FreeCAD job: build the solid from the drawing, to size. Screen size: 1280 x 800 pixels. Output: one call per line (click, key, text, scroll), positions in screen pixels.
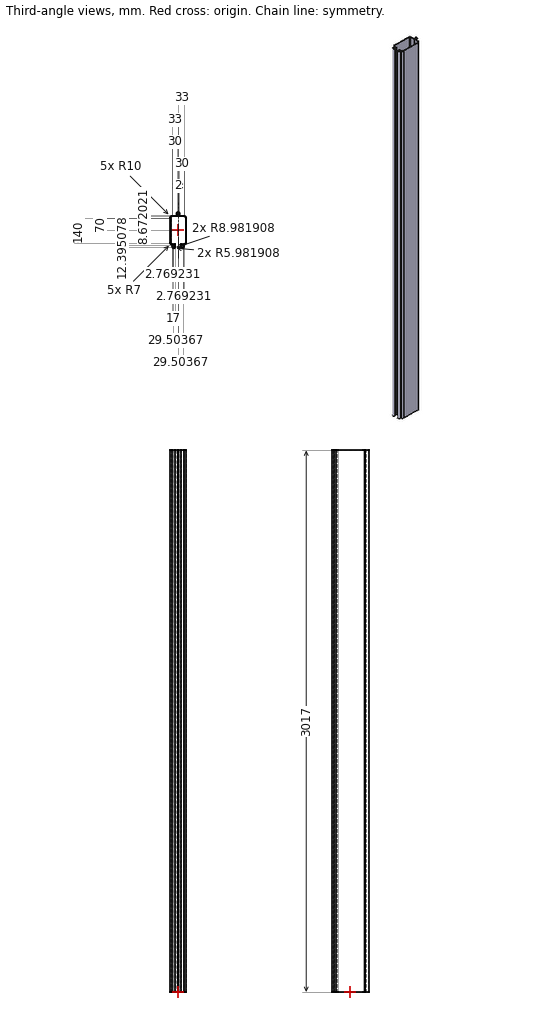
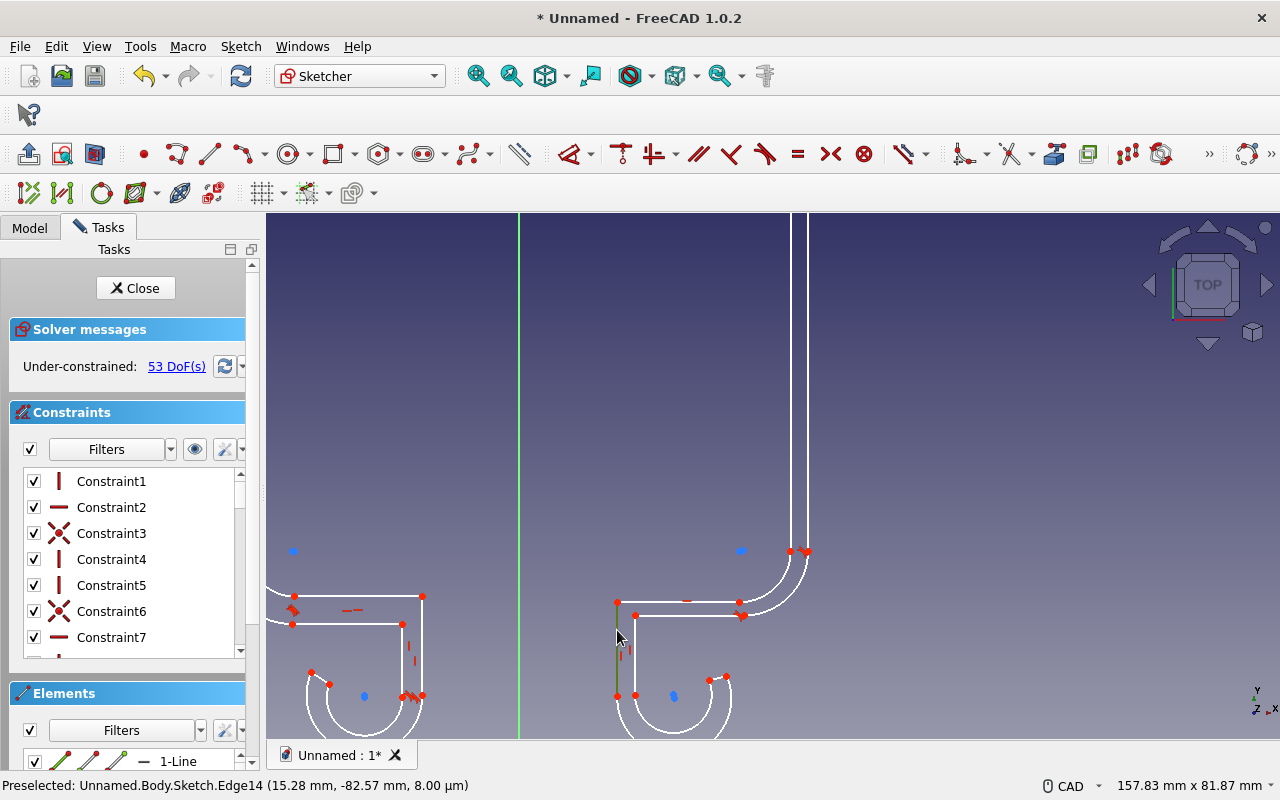
scroll(765, 600, down, 7)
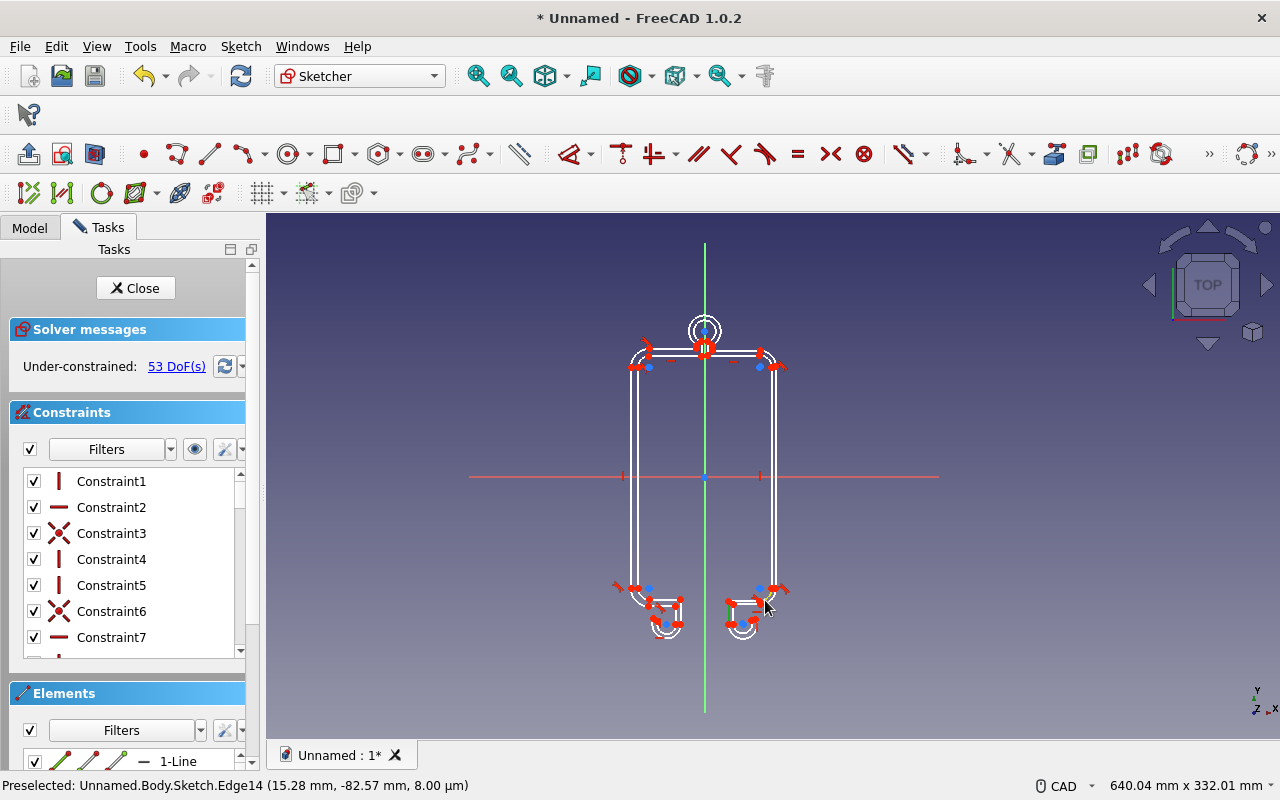
scroll(736, 637, up, 5)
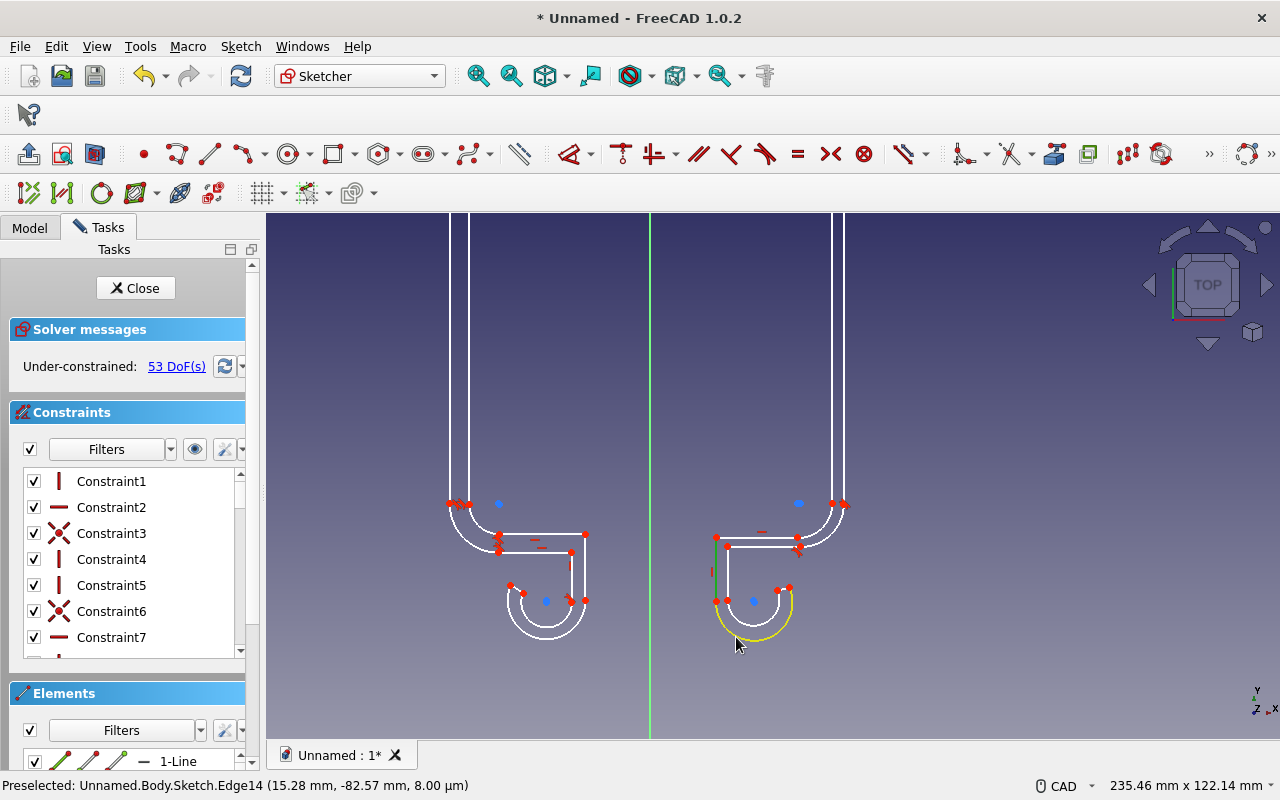
click(735, 635)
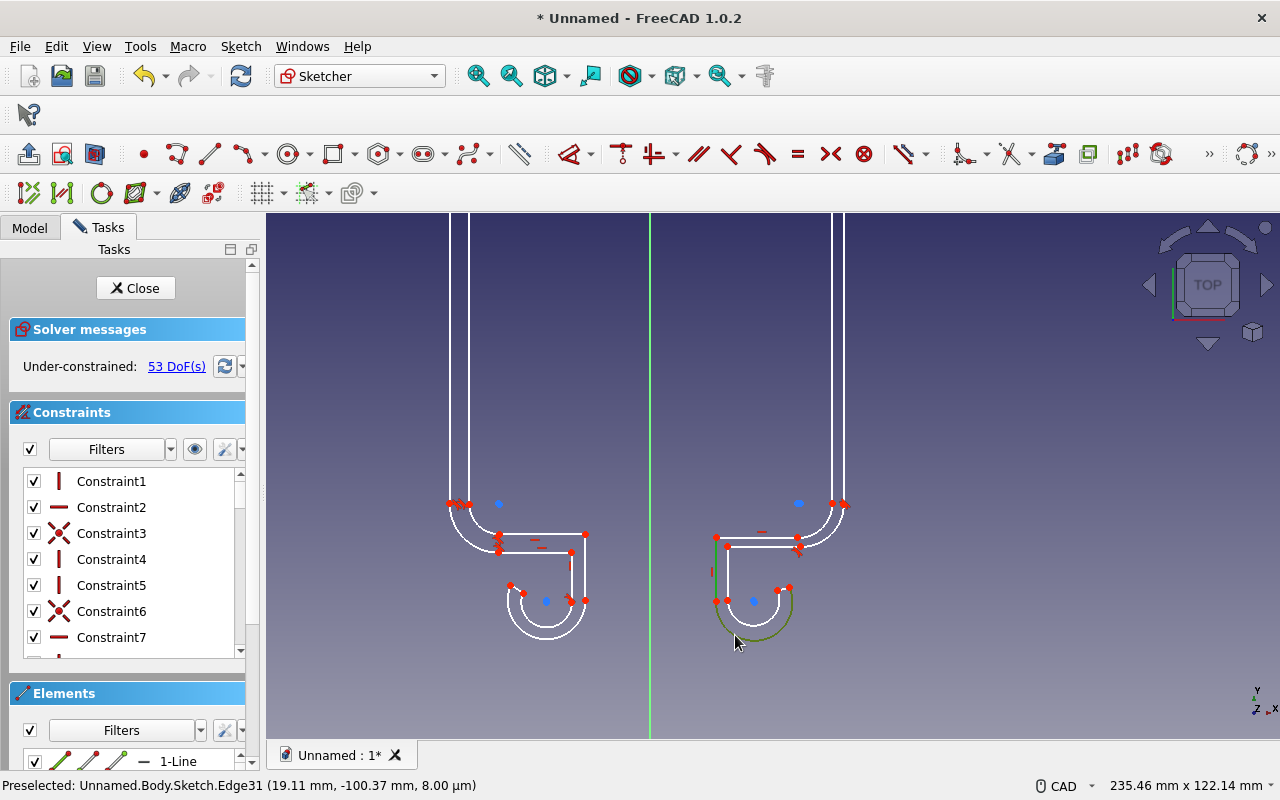
click(765, 154)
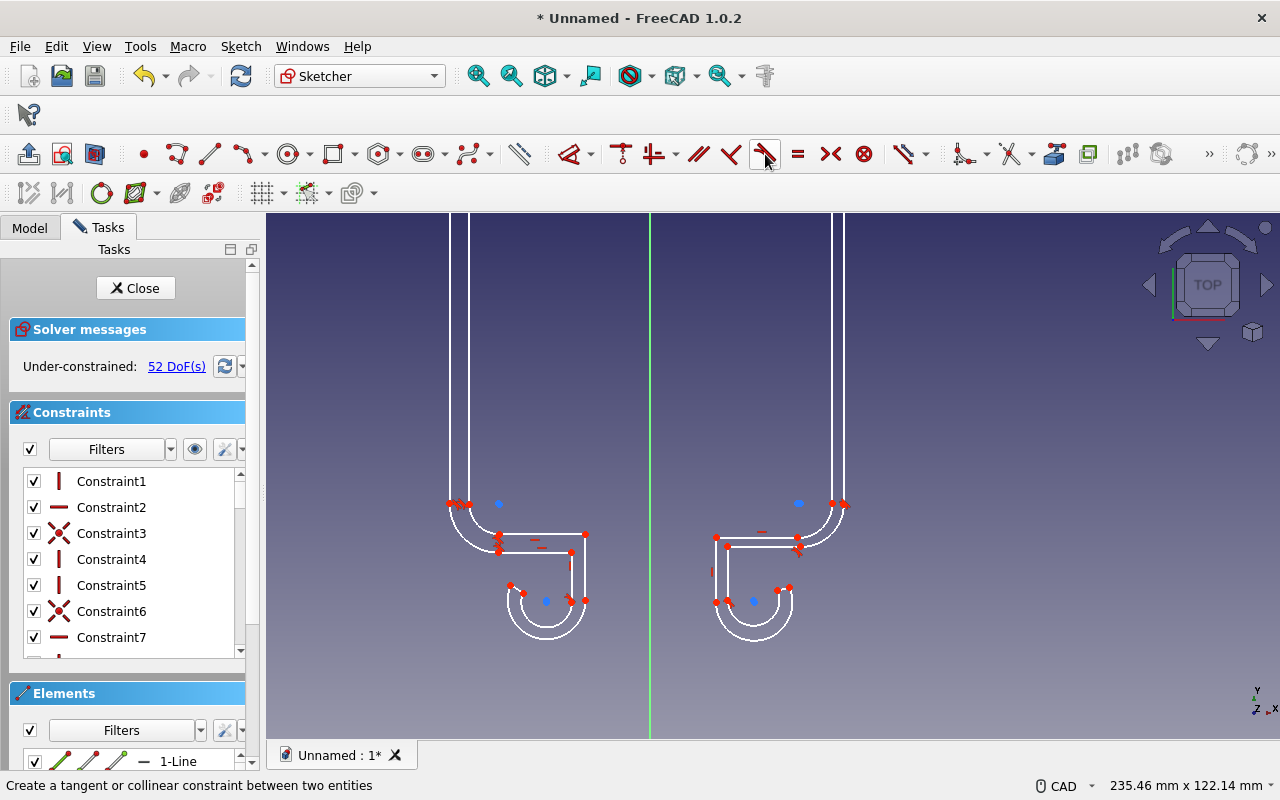
click(728, 585)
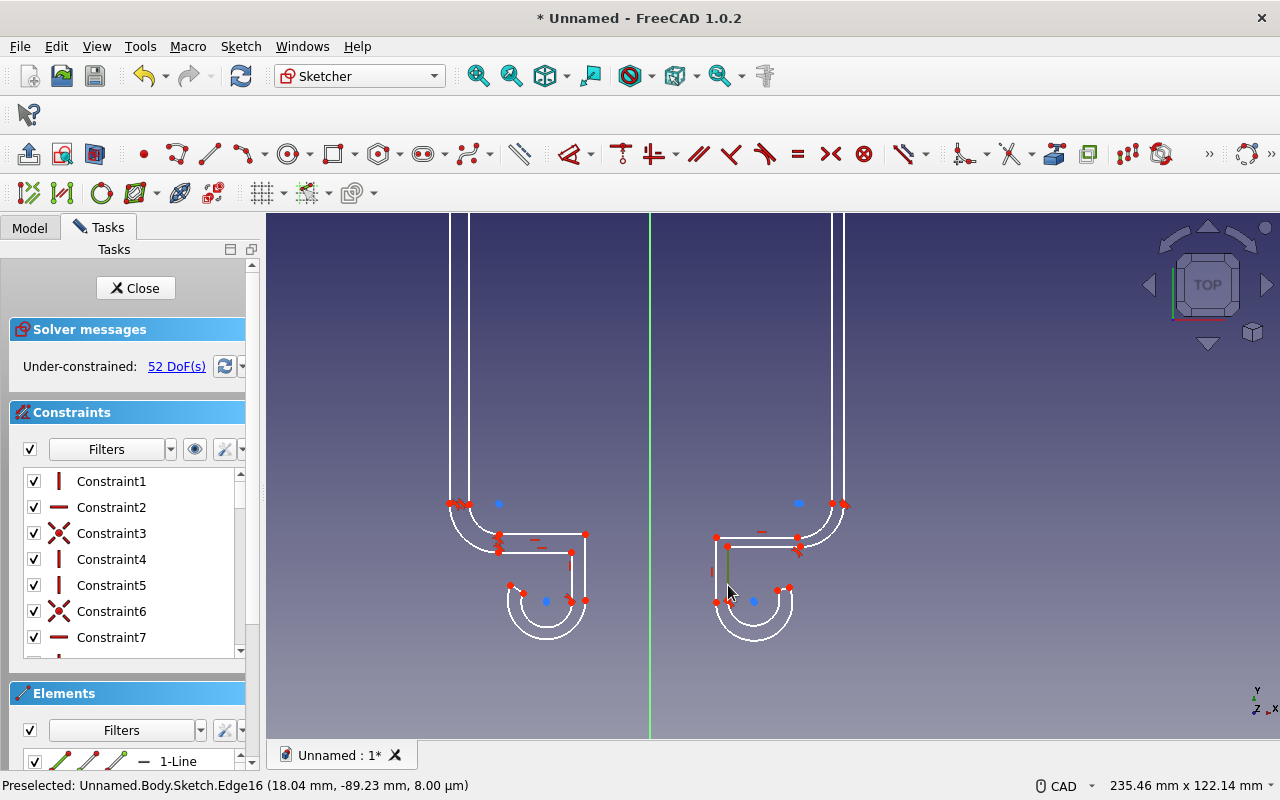
click(741, 623)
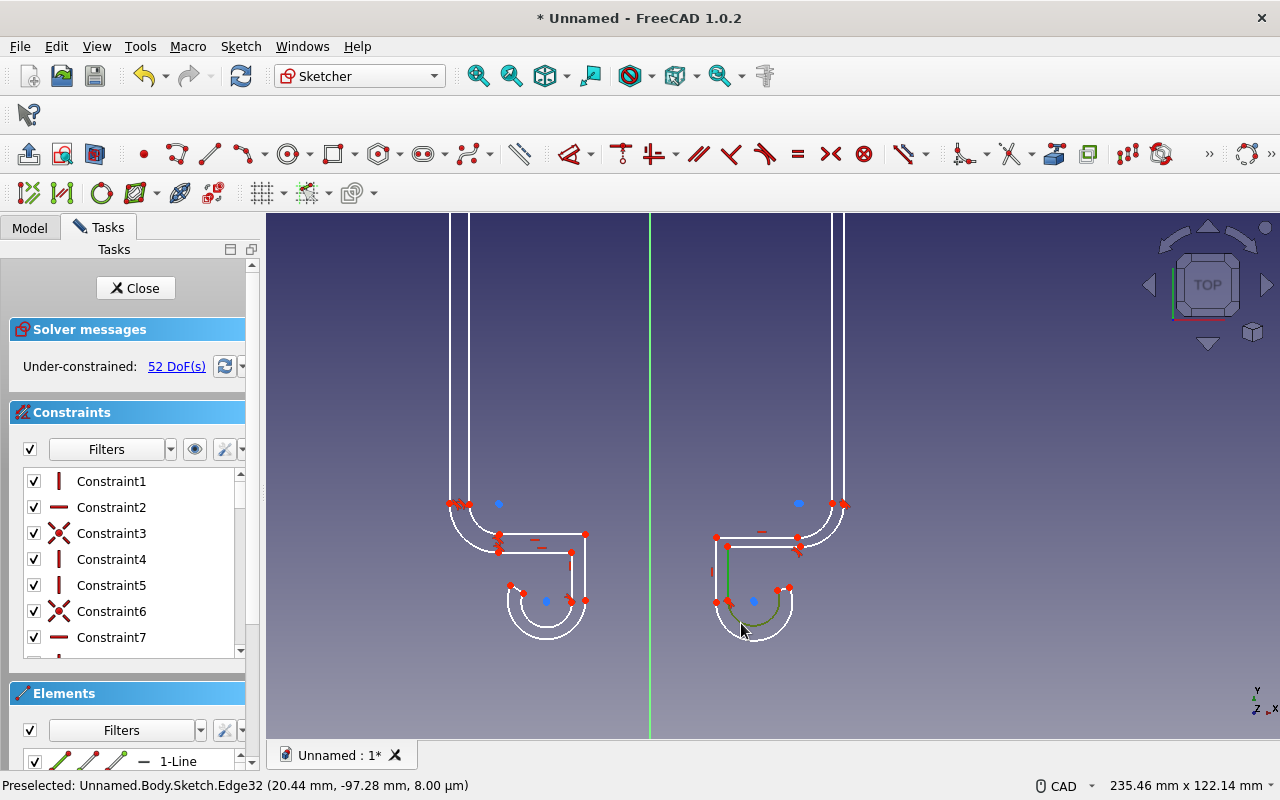
click(765, 154)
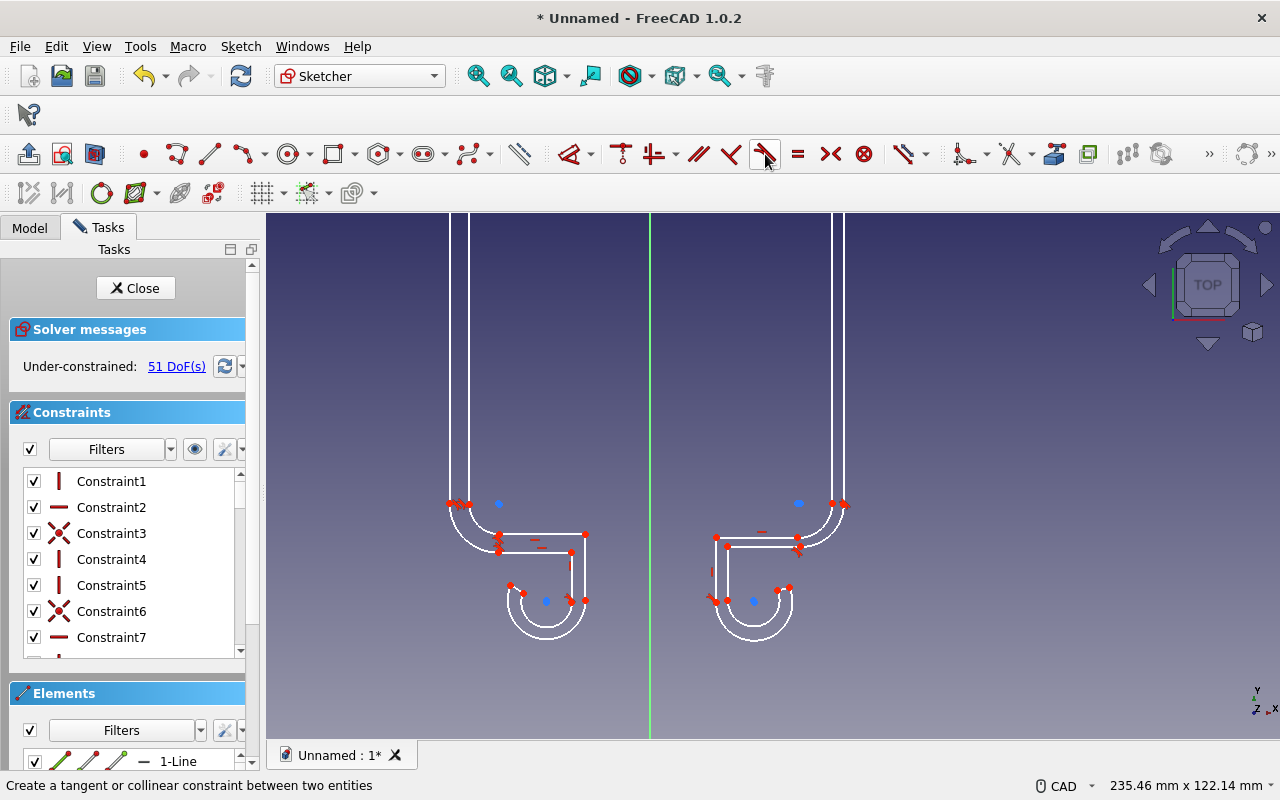
scroll(750, 547, up, 3)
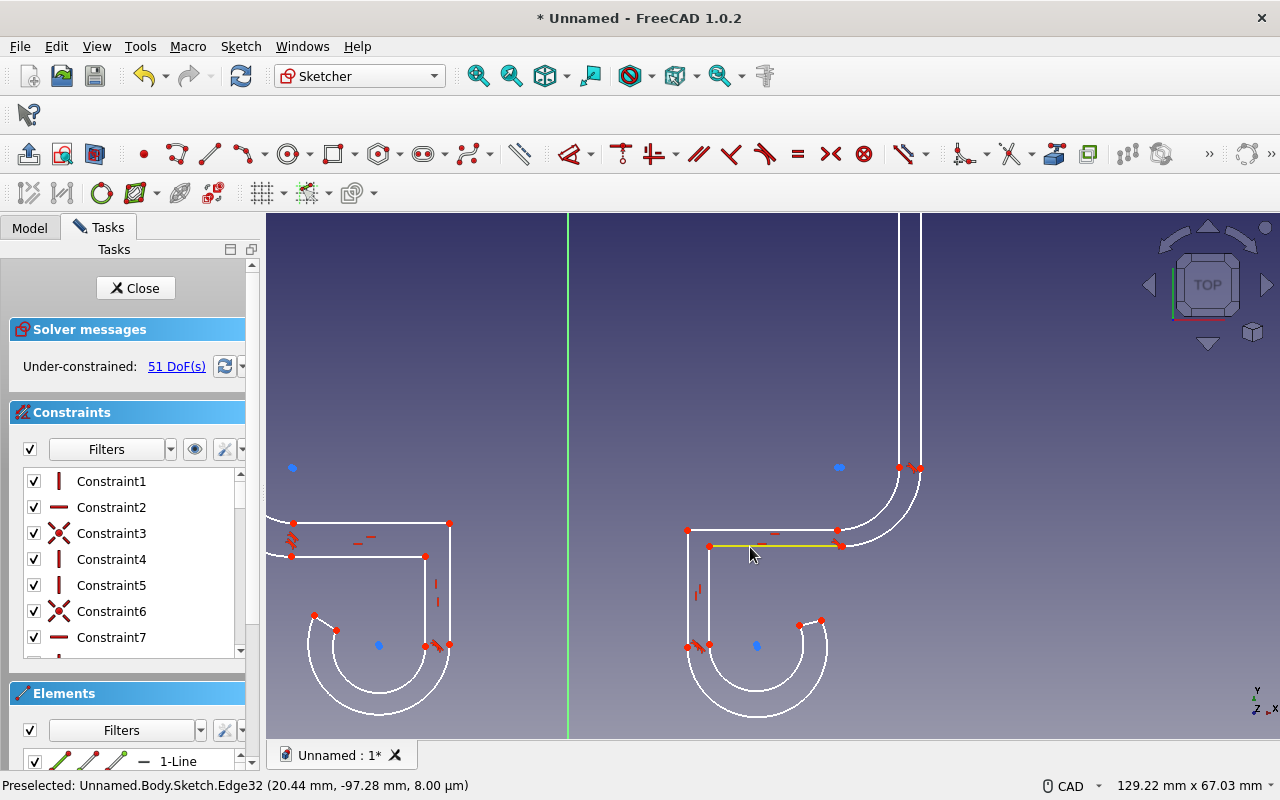
click(749, 546)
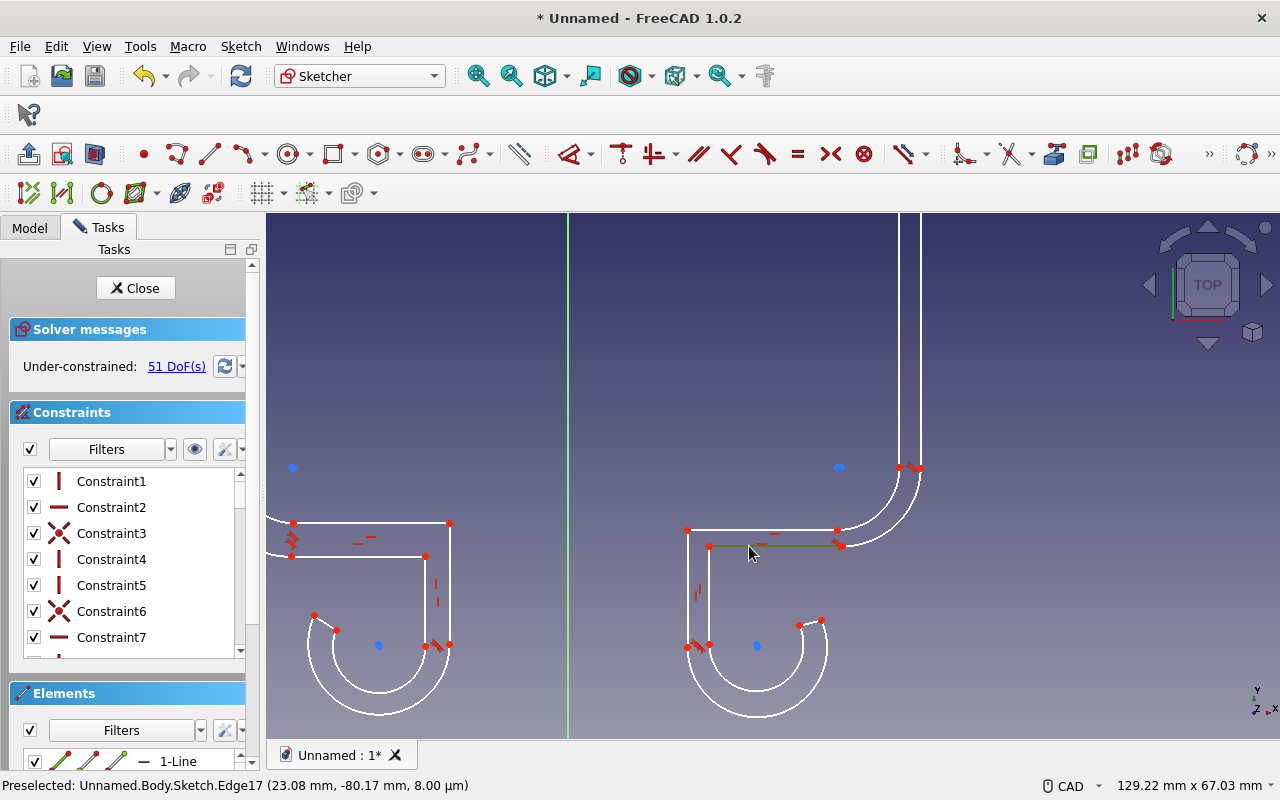
click(878, 538)